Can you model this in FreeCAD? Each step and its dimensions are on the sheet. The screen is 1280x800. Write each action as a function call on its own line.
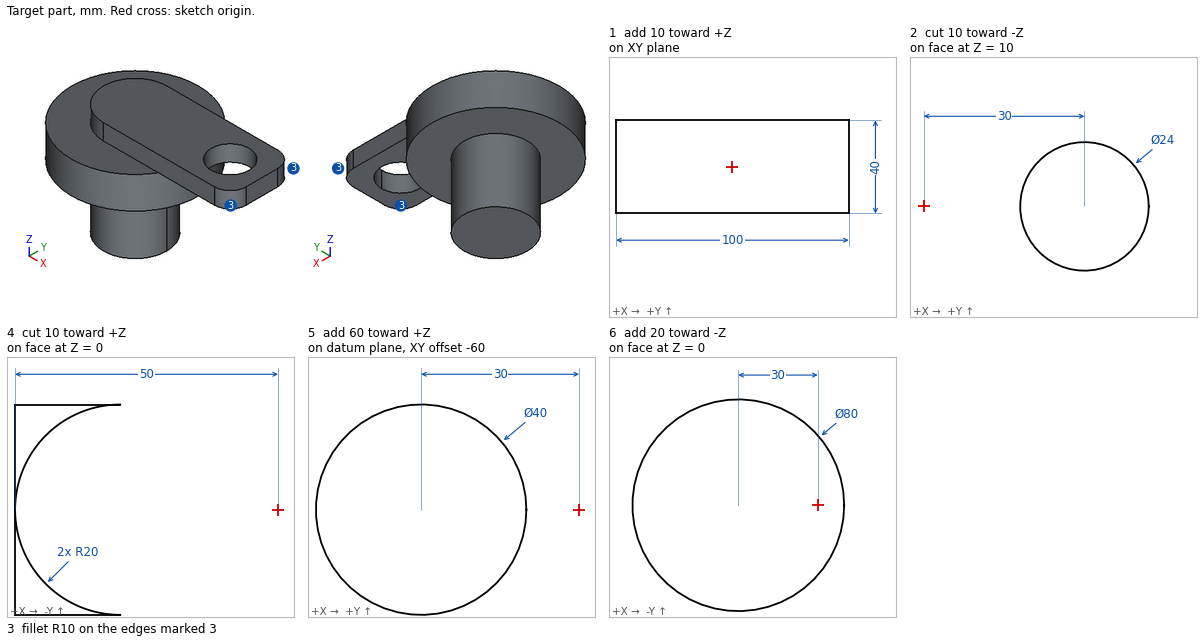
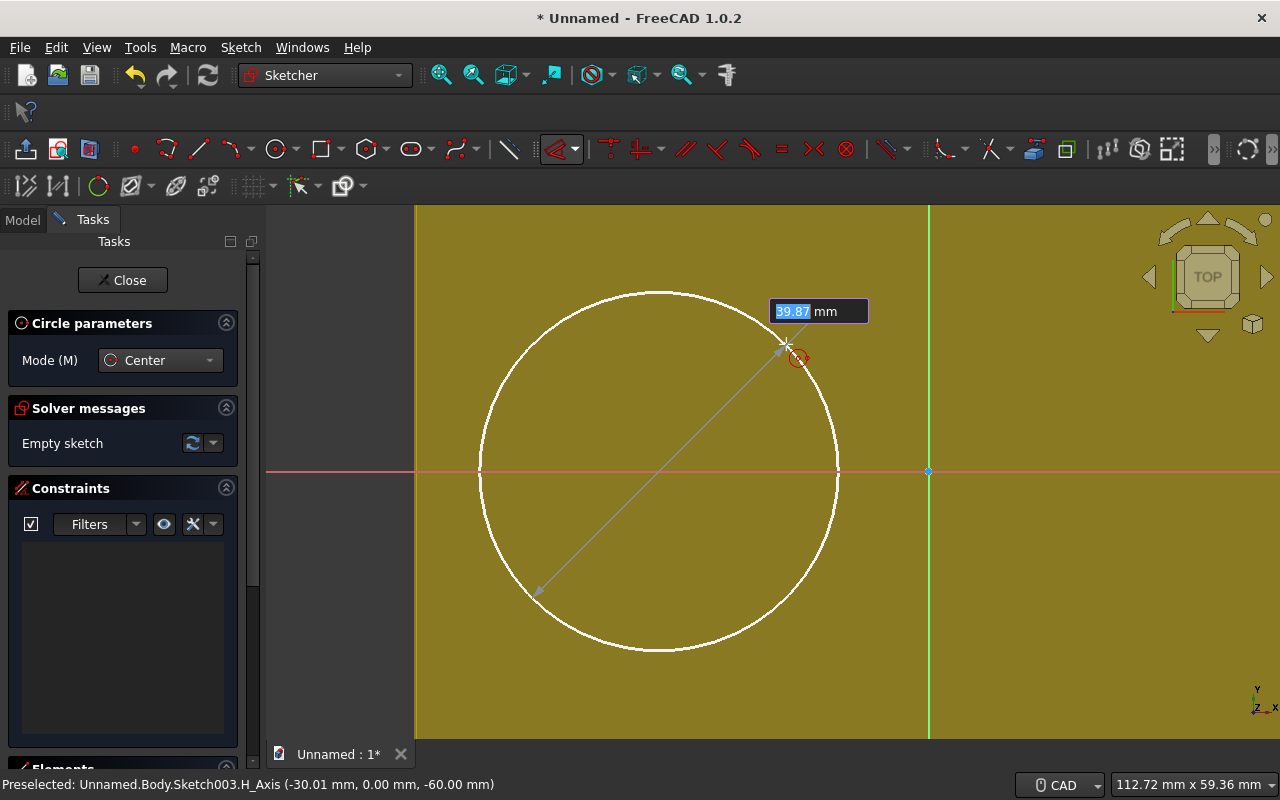
text(40)
key(Return)
key(Escape)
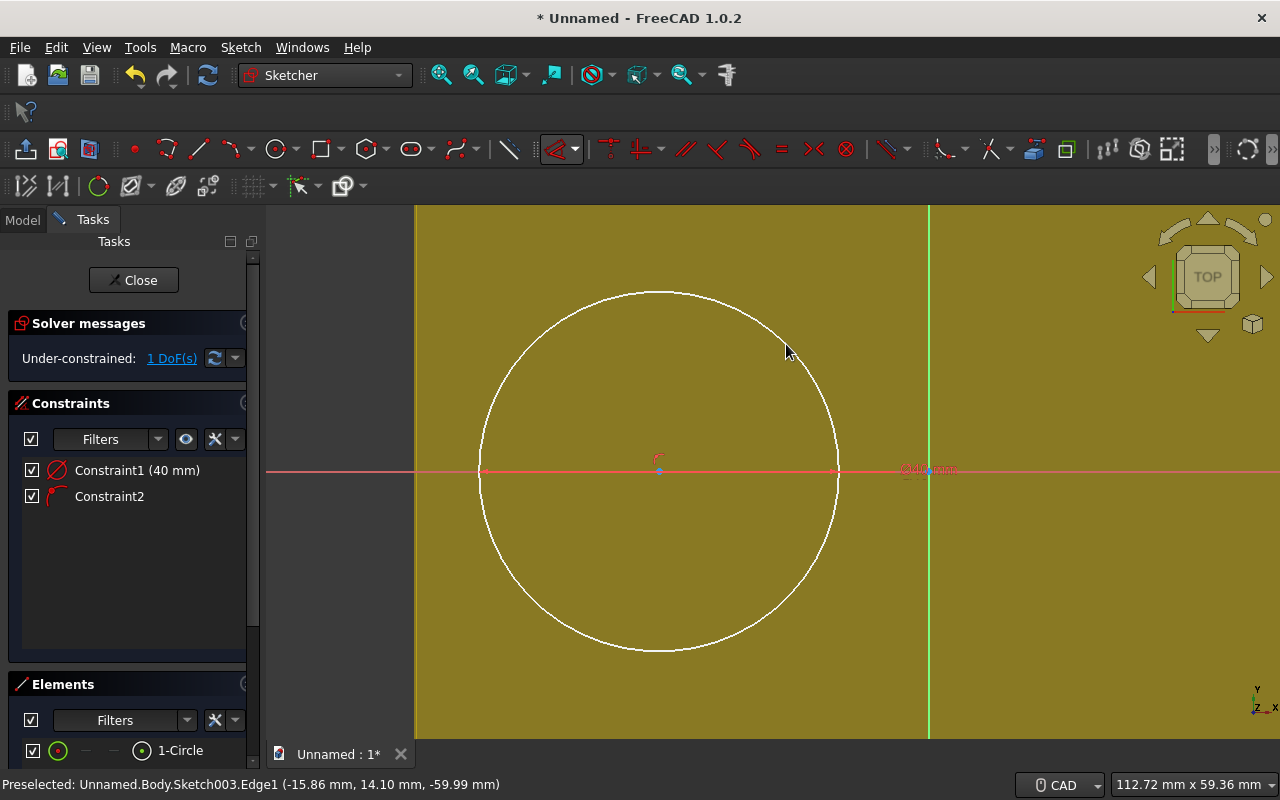
click(659, 472)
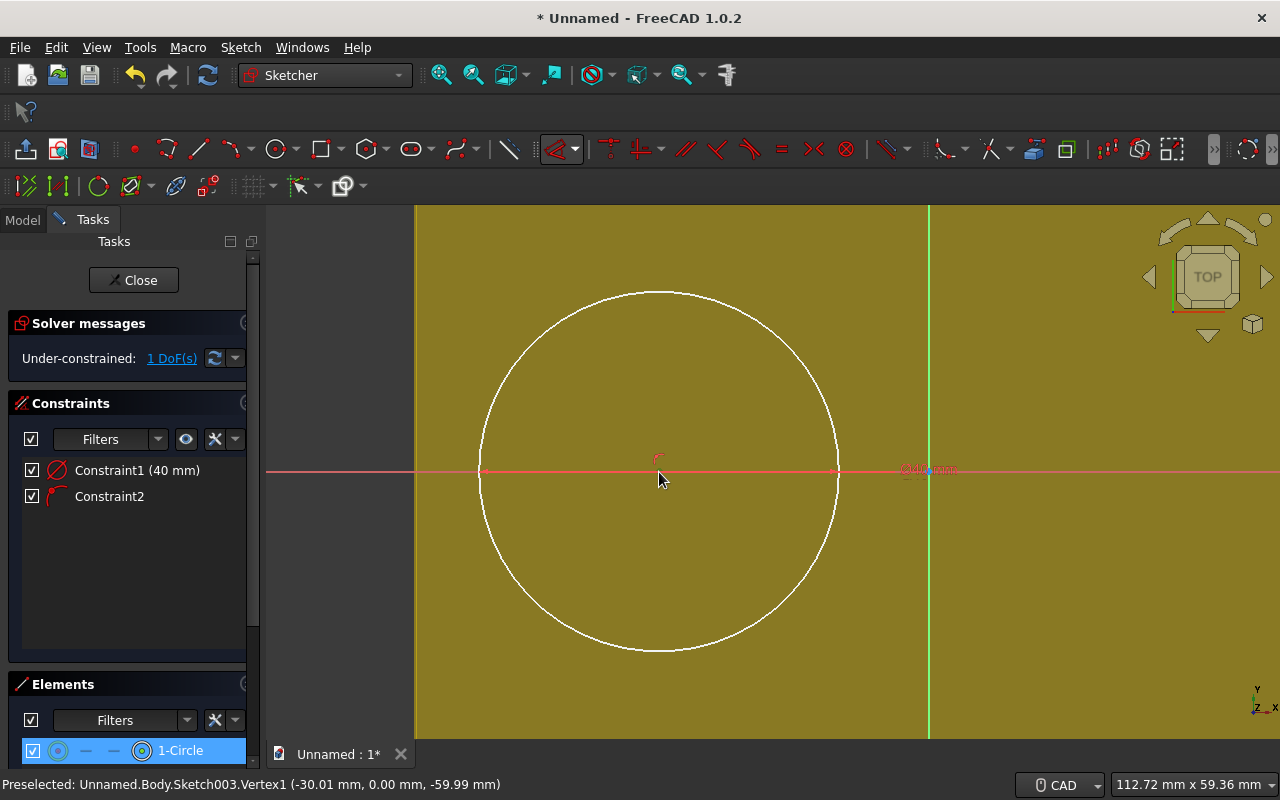
key(l)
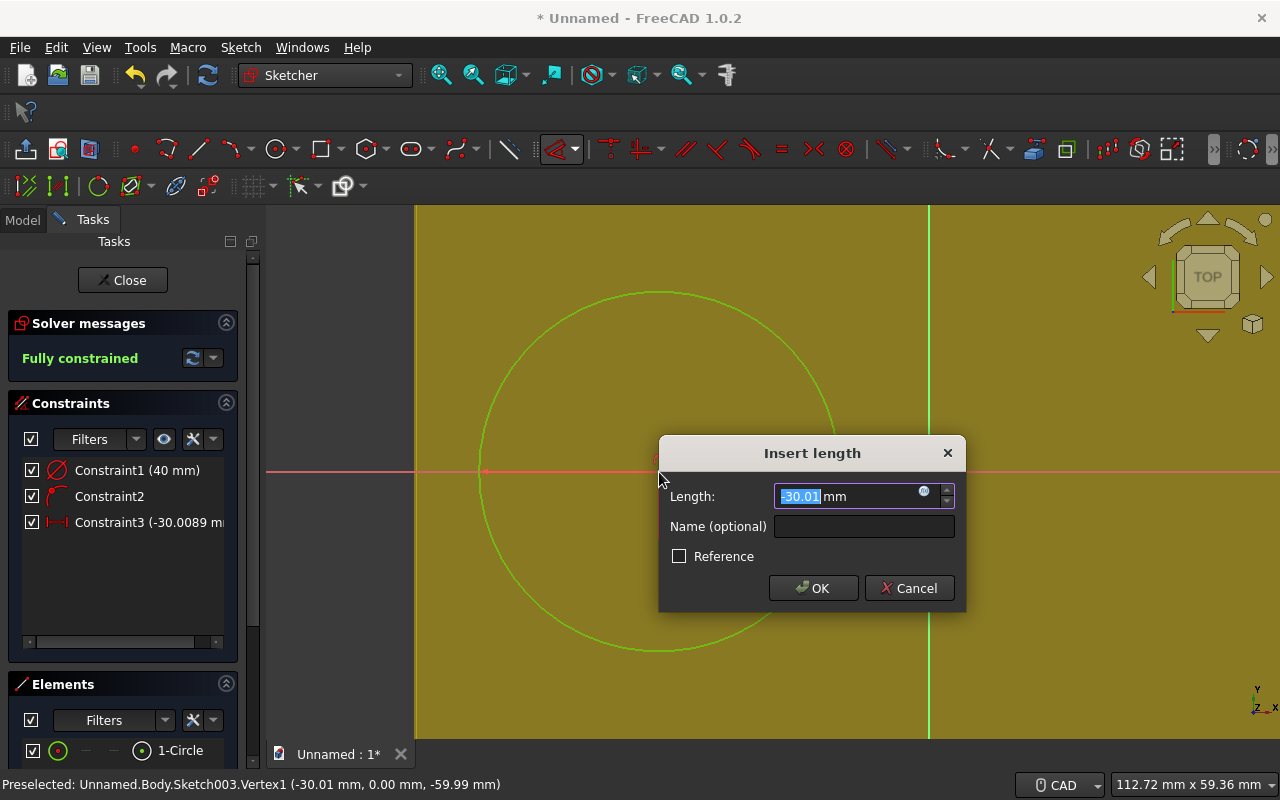
text(-30)
key(Return)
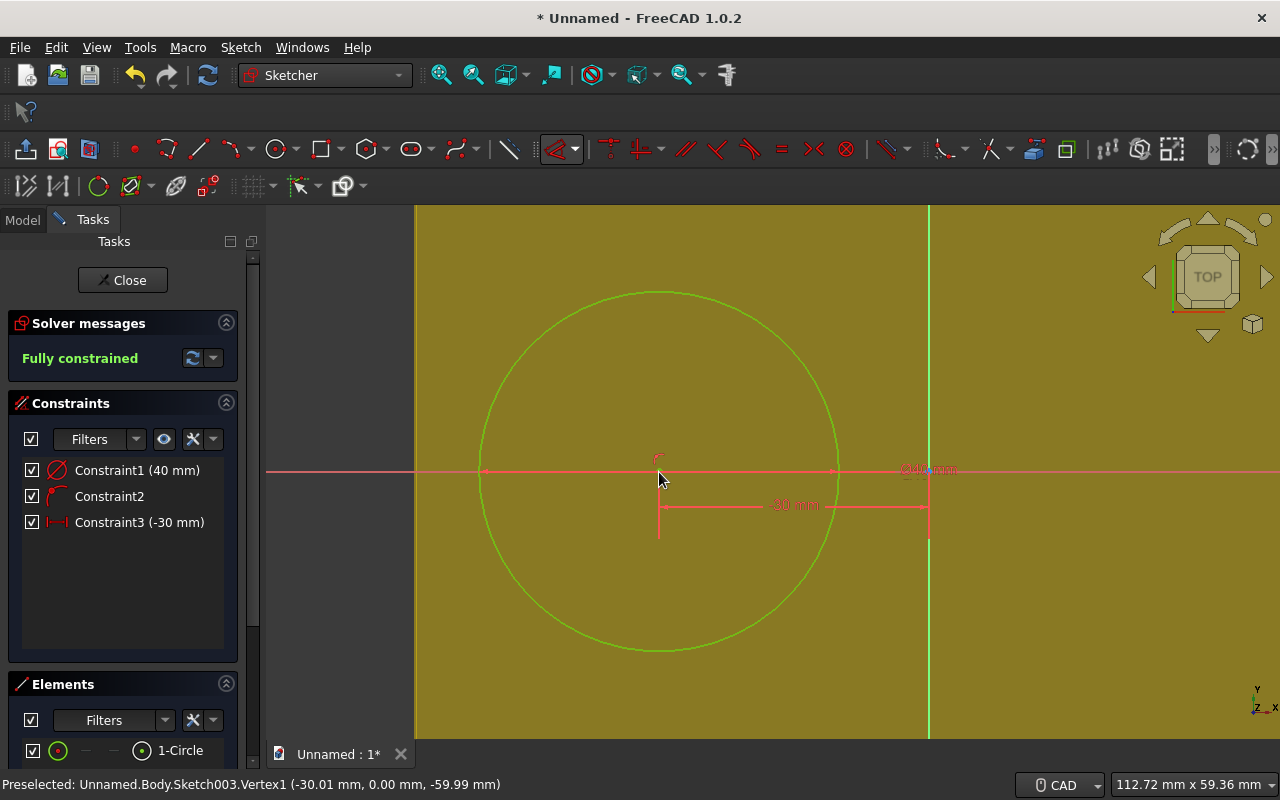
click(123, 280)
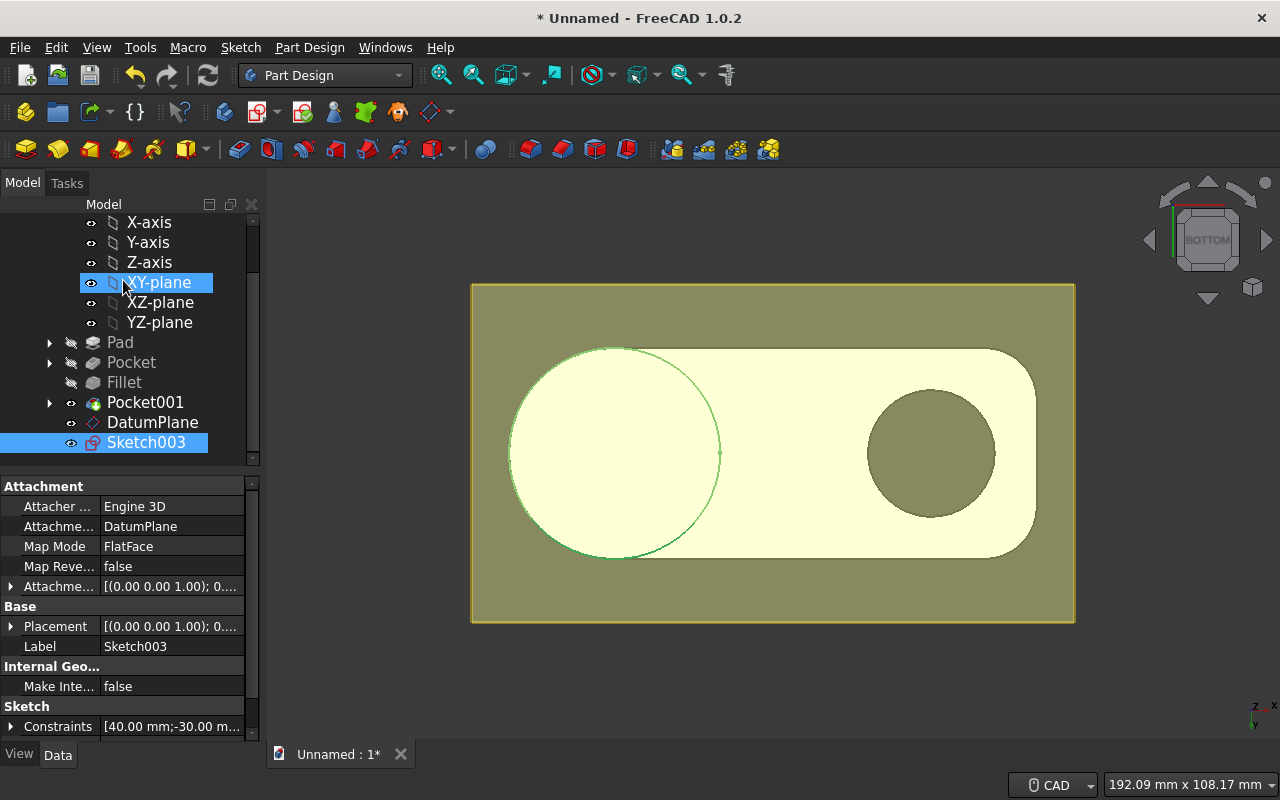
click(26, 150)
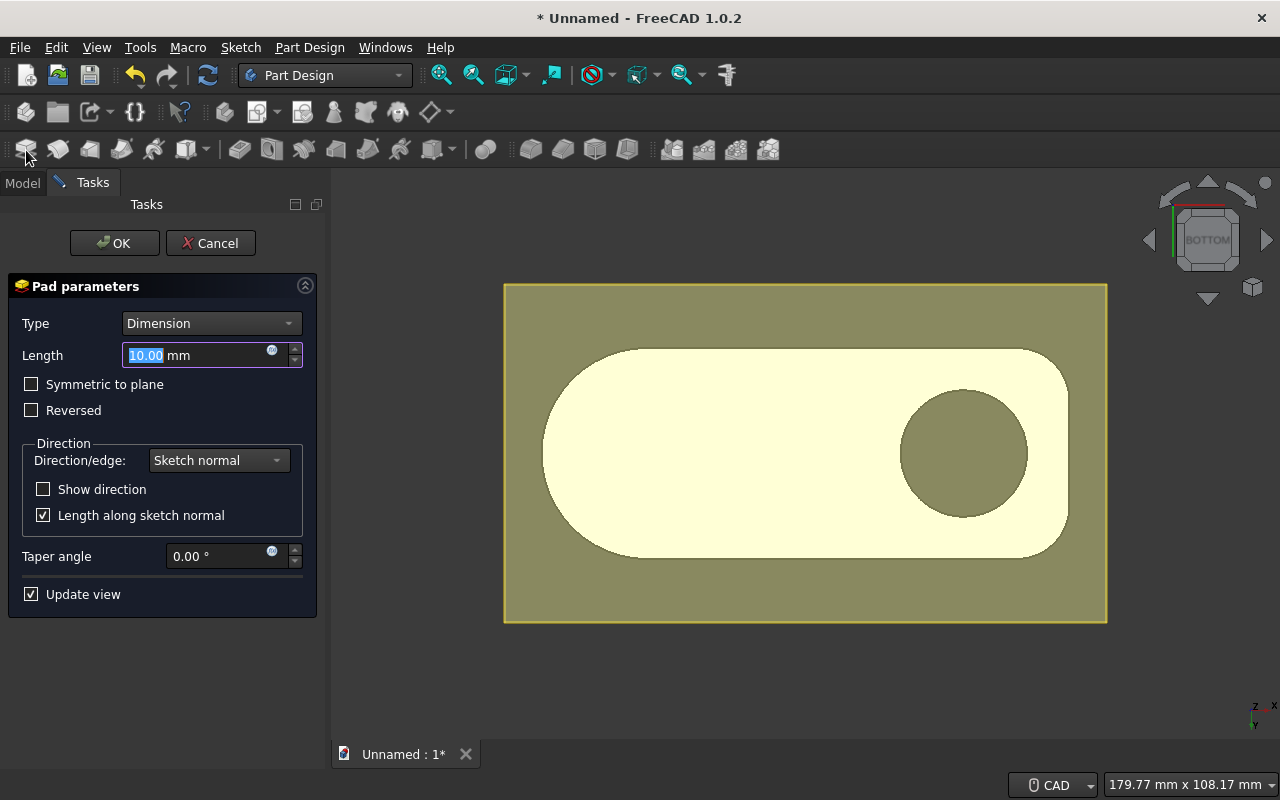
text(60)
key(Tab)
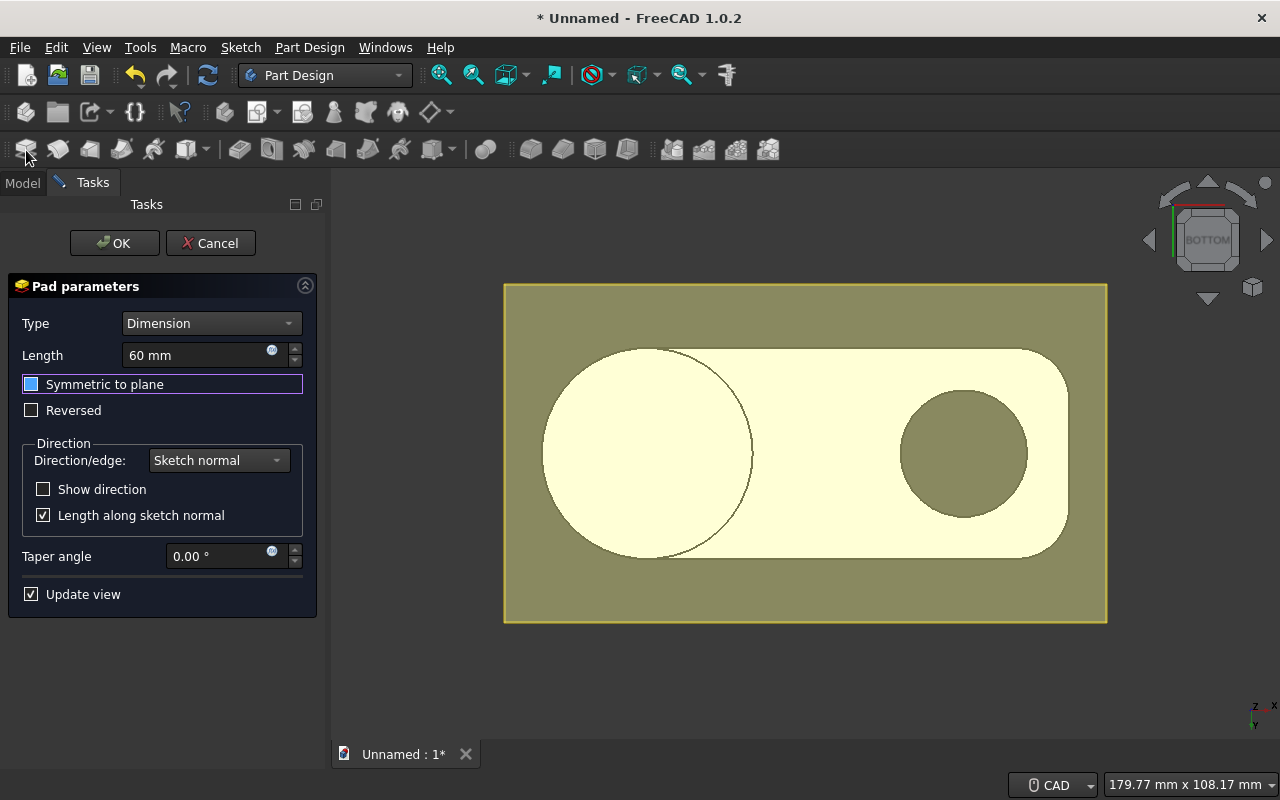
click(115, 243)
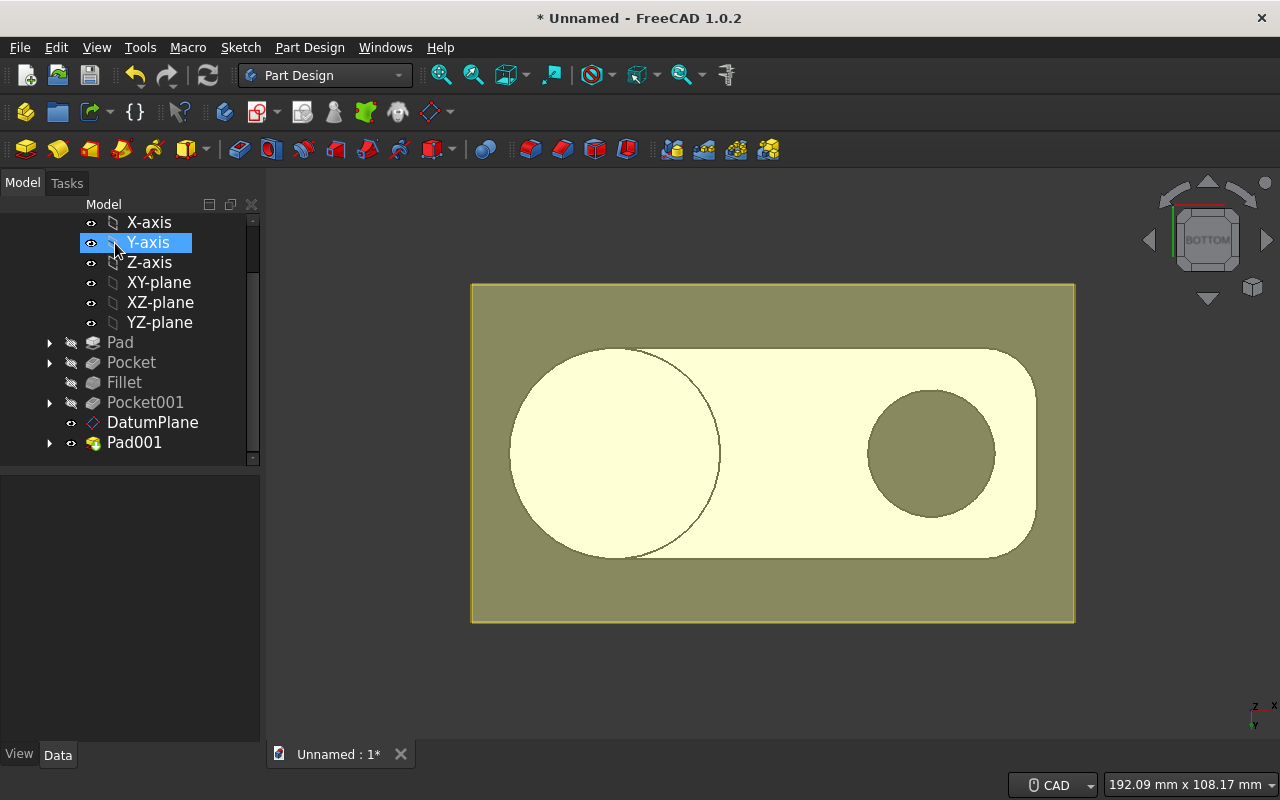
click(116, 423)
key(space)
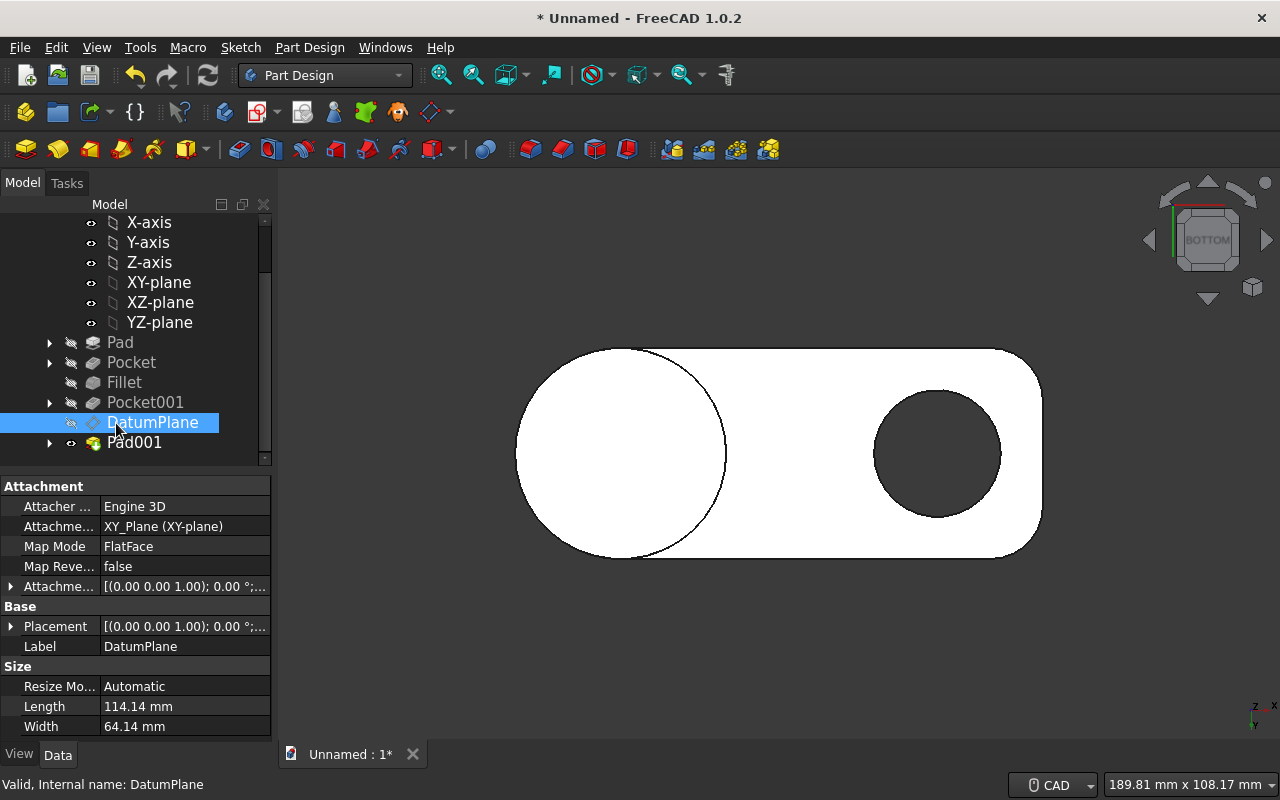
click(771, 483)